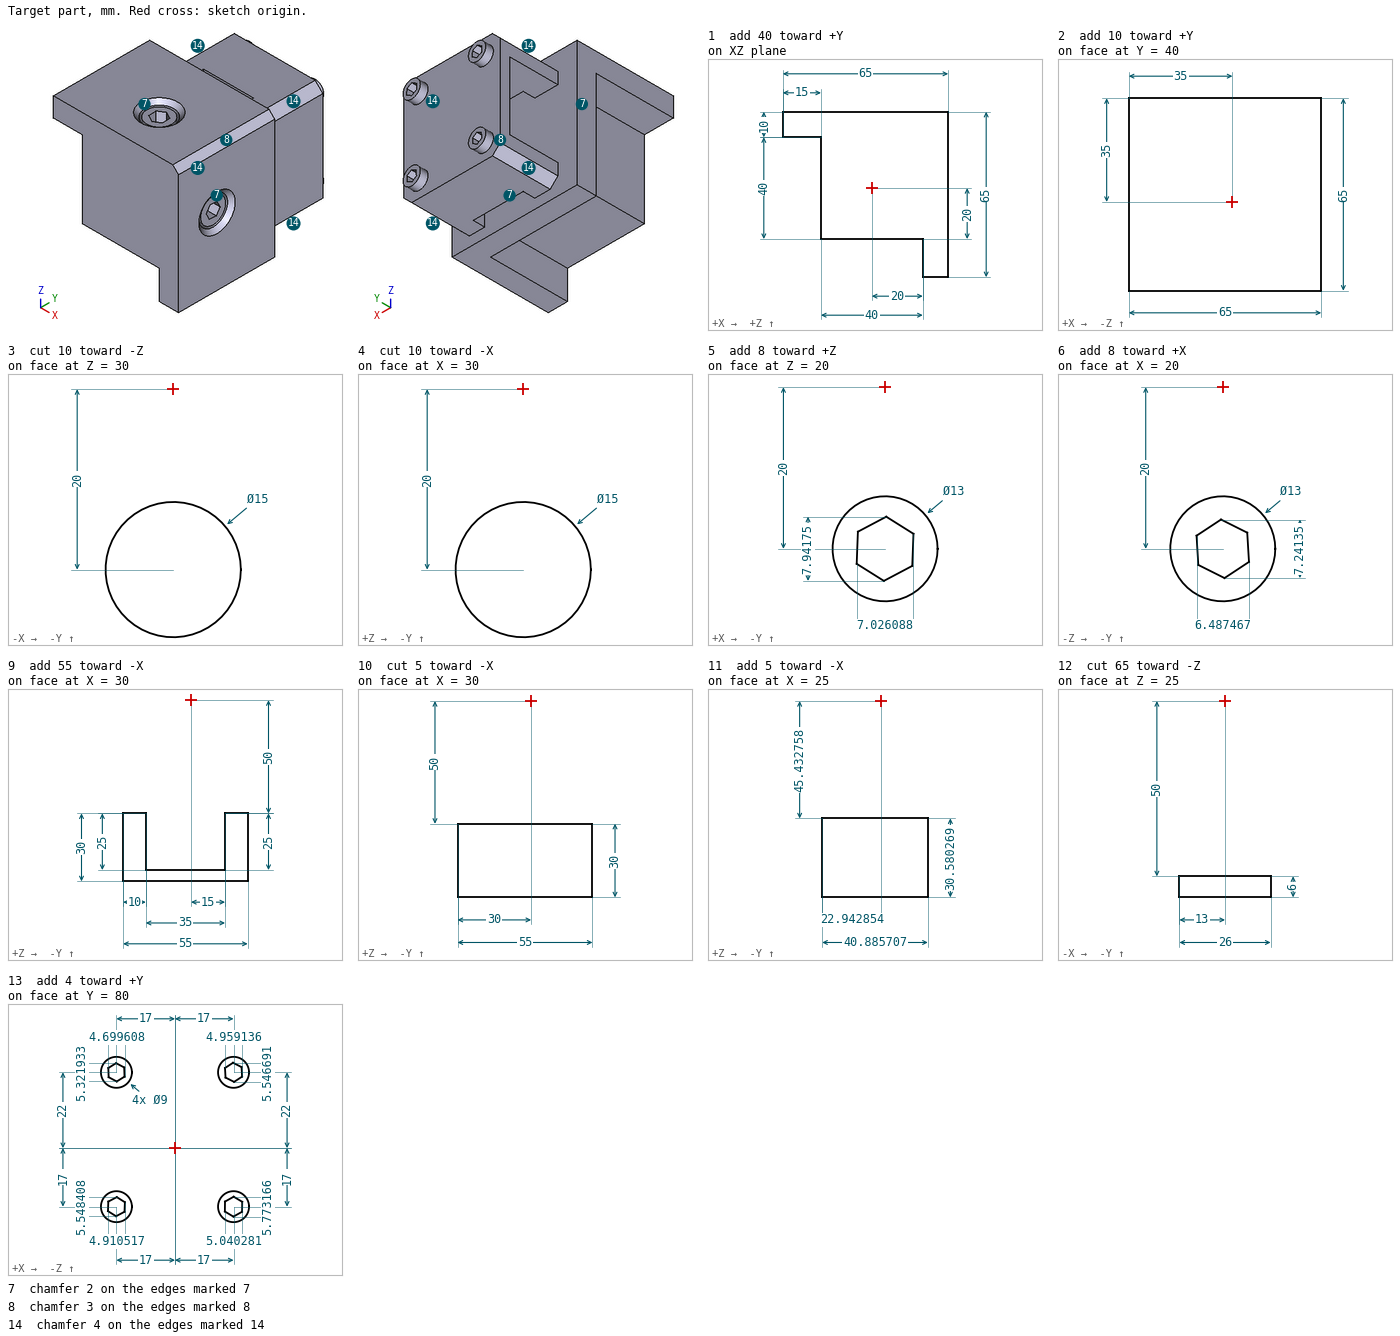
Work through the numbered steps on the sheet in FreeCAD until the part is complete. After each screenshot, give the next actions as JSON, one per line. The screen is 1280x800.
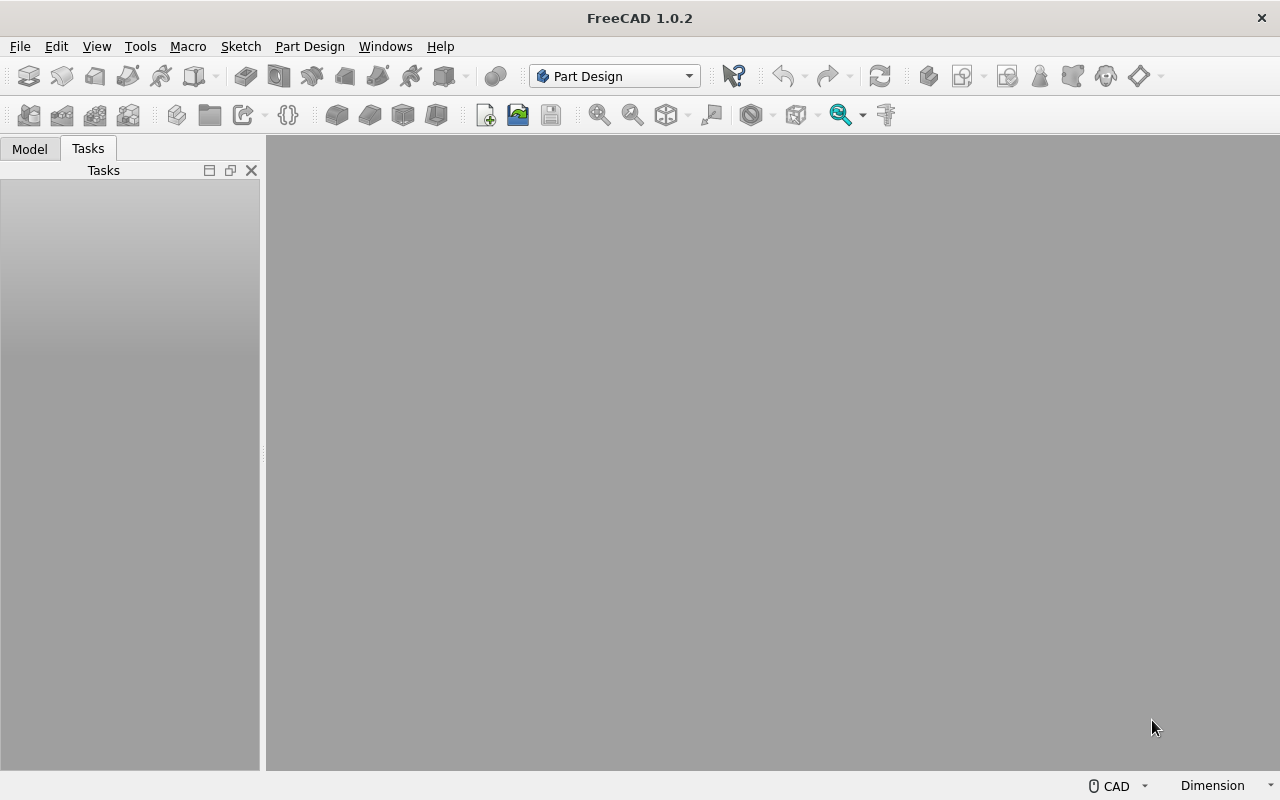
{"action": "left_click", "coordinate": [485, 116]}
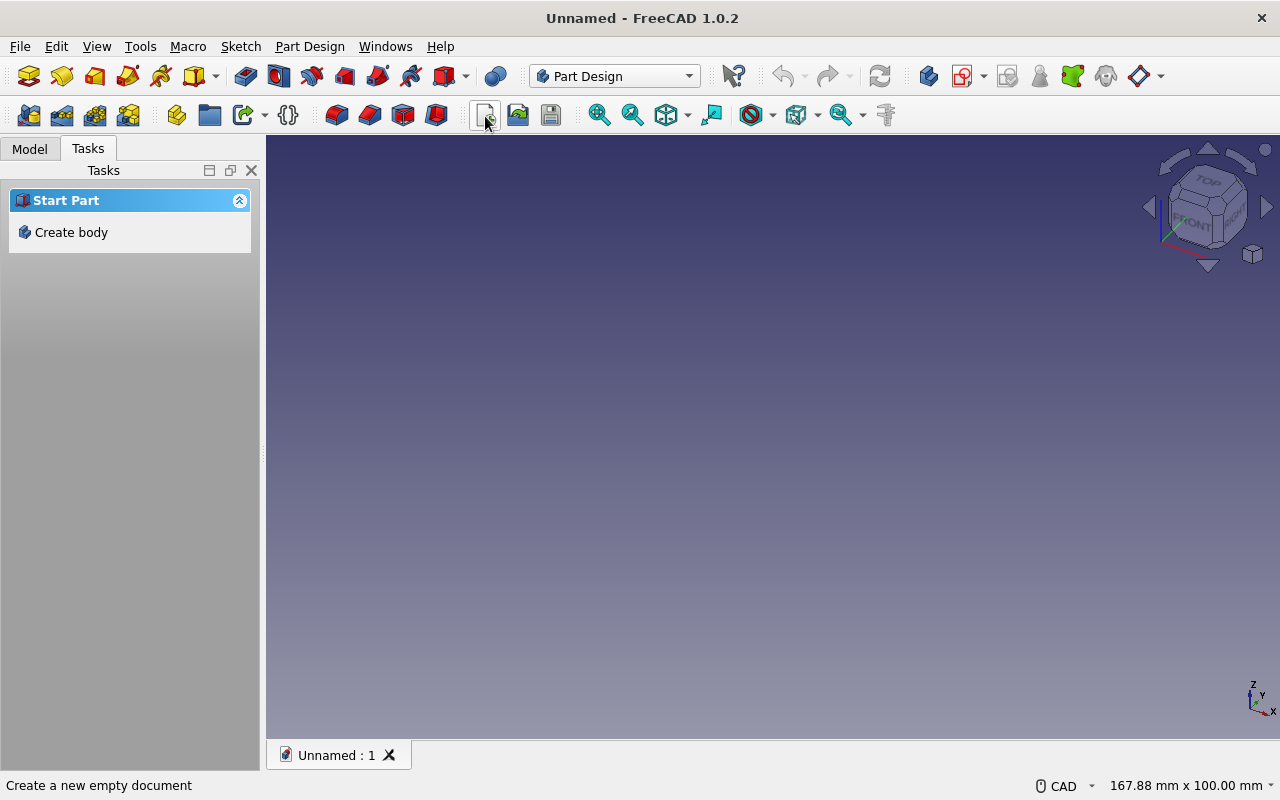
{"action": "left_click", "coordinate": [962, 76]}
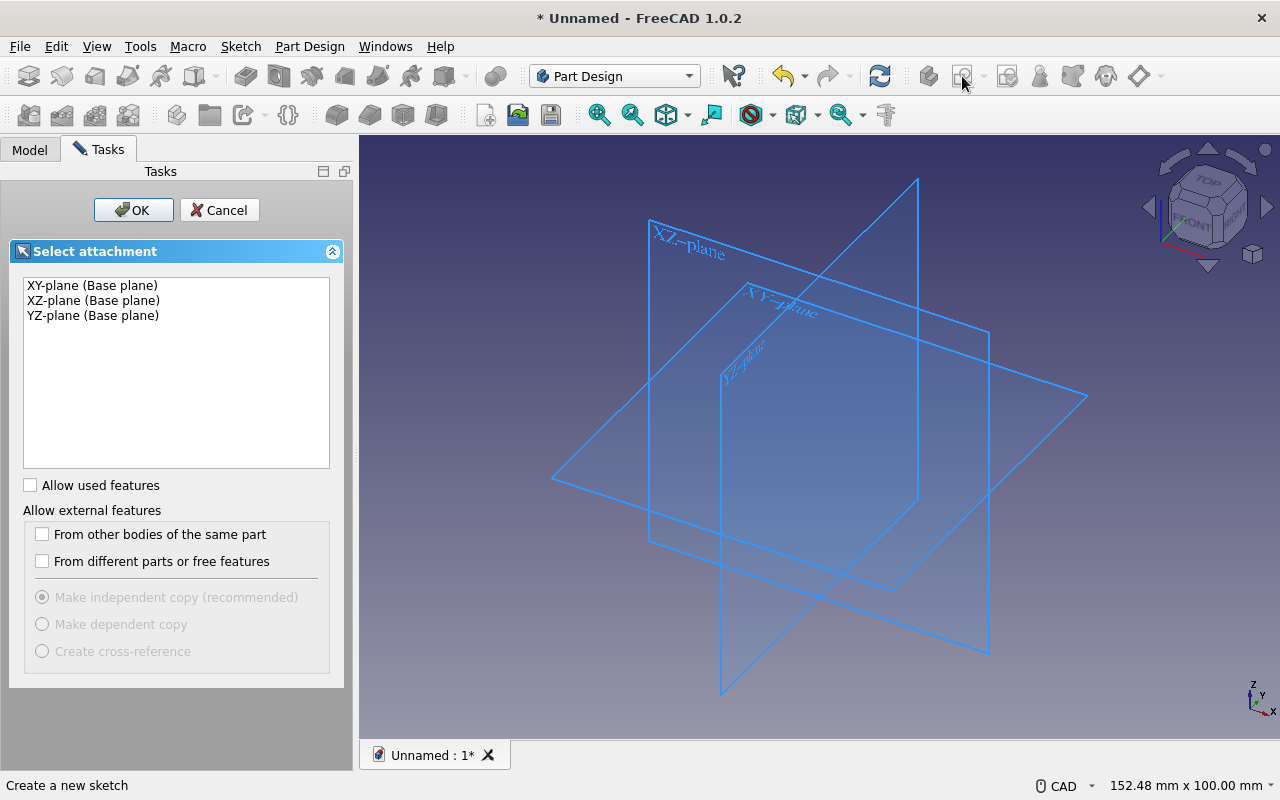
{"action": "left_click", "coordinate": [84, 300]}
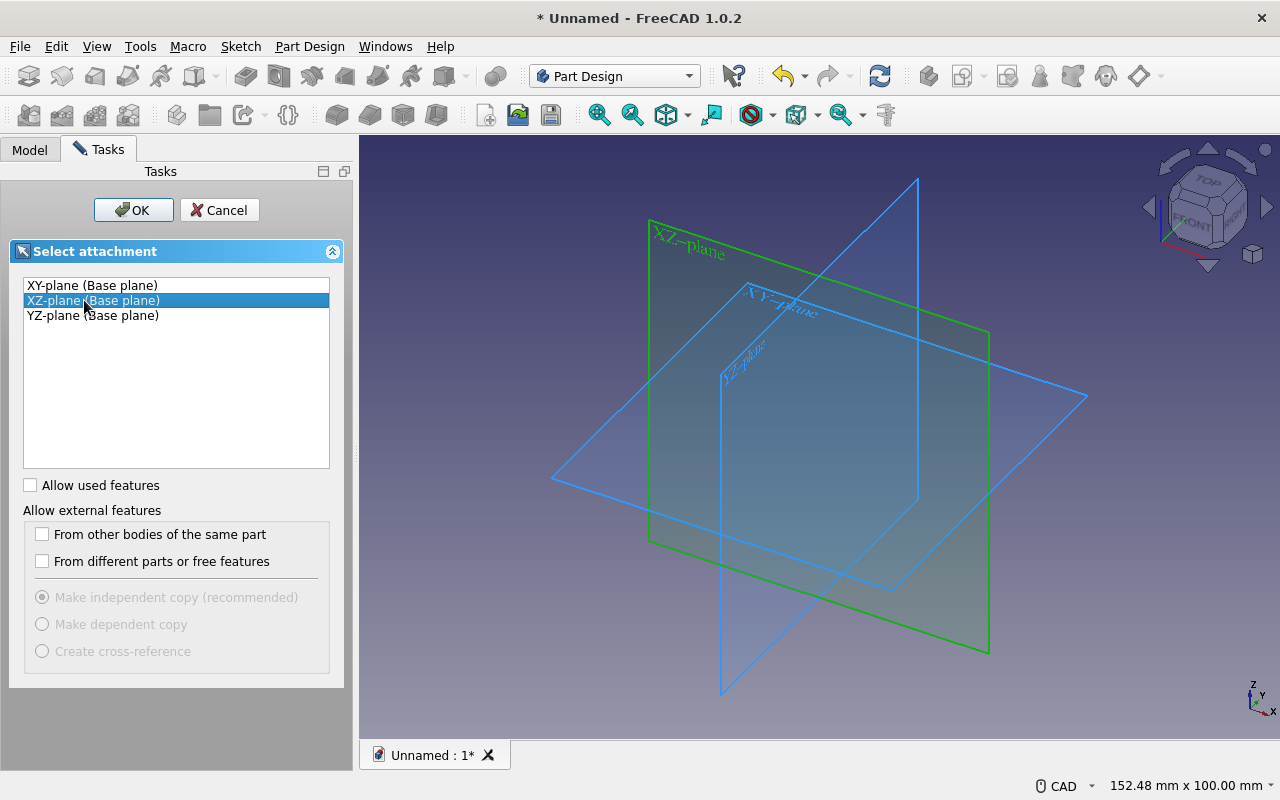
{"action": "left_click", "coordinate": [134, 210]}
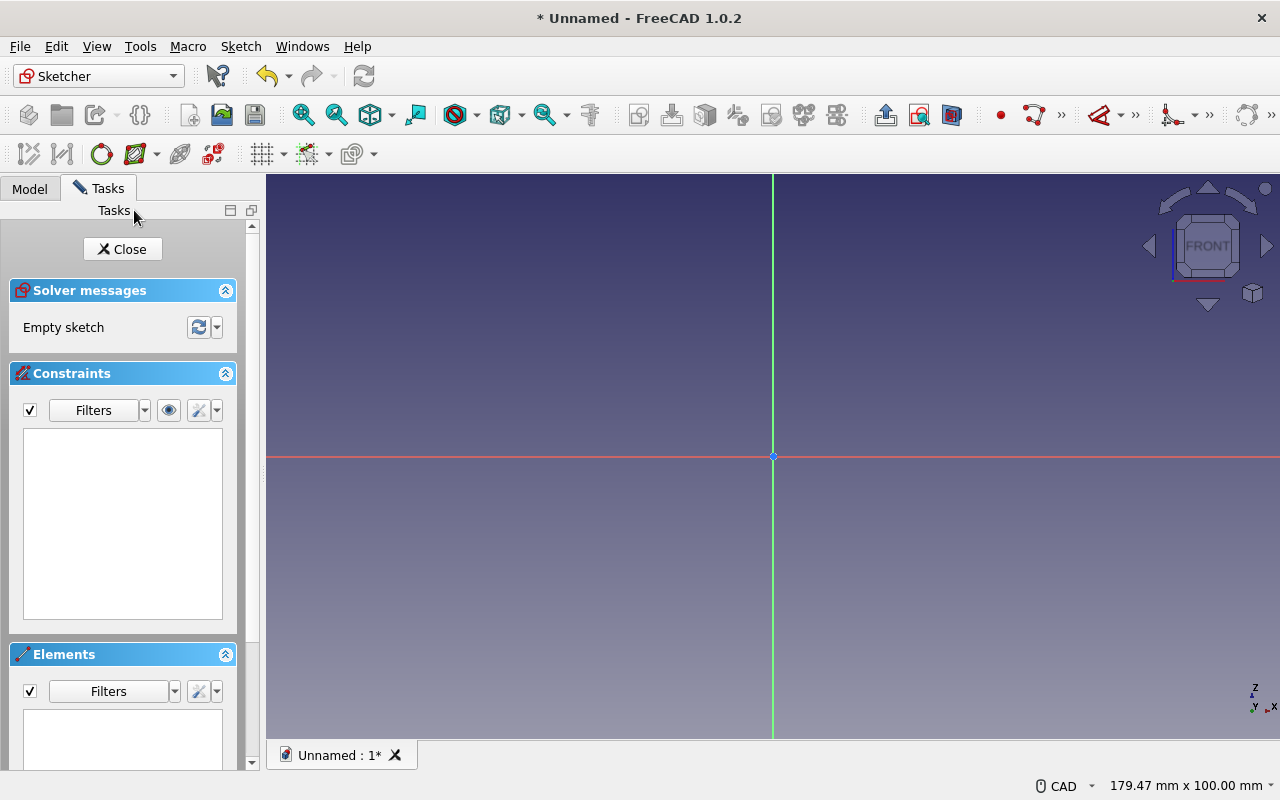
{"action": "left_click", "coordinate": [1034, 116]}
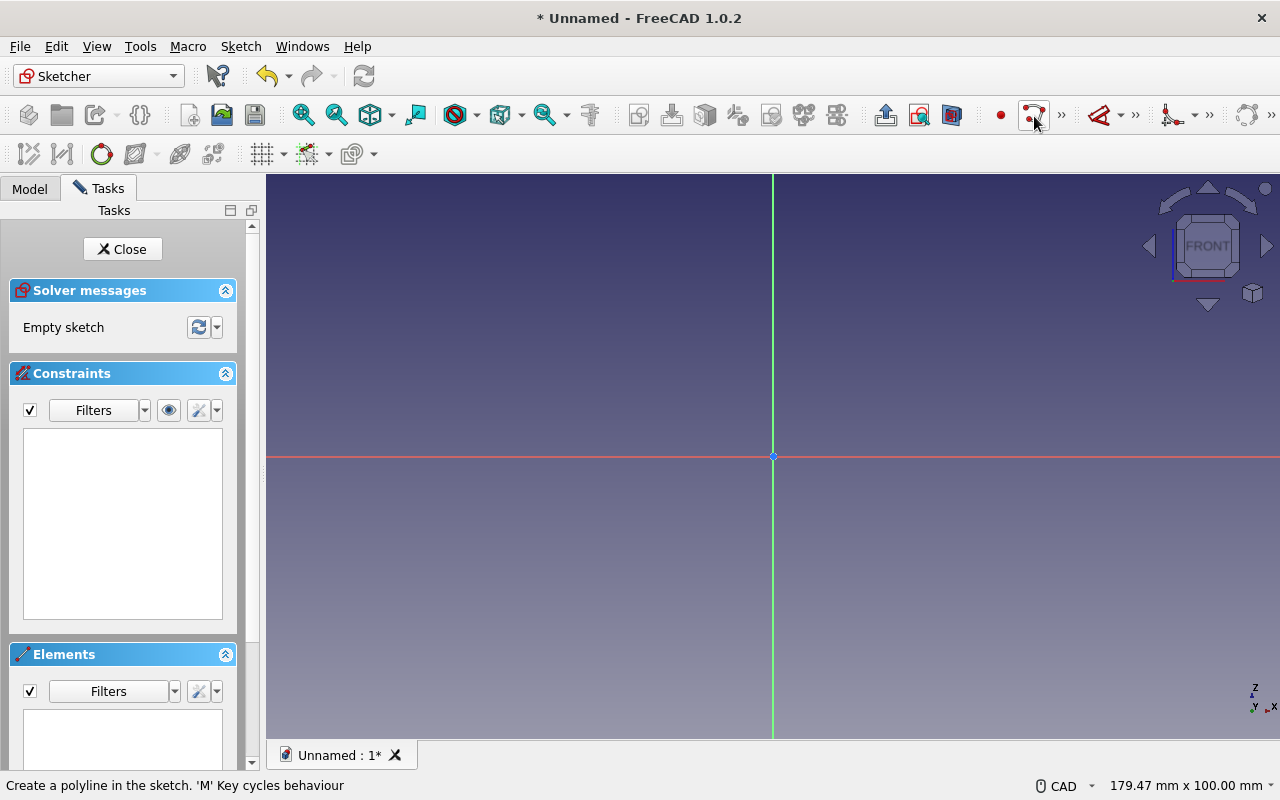
{"action": "left_click", "coordinate": [886, 570]}
{"action": "left_click", "coordinate": [660, 570]}
{"action": "left_click", "coordinate": [660, 344]}
{"action": "left_click", "coordinate": [575, 344]}
{"action": "left_click", "coordinate": [575, 287]}
{"action": "left_click", "coordinate": [942, 287]}
{"action": "left_click", "coordinate": [942, 654]}
{"action": "left_click", "coordinate": [886, 654]}
{"action": "left_click", "coordinate": [886, 571]}
{"action": "key", "text": "Escape"}
{"action": "key", "text": "Escape"}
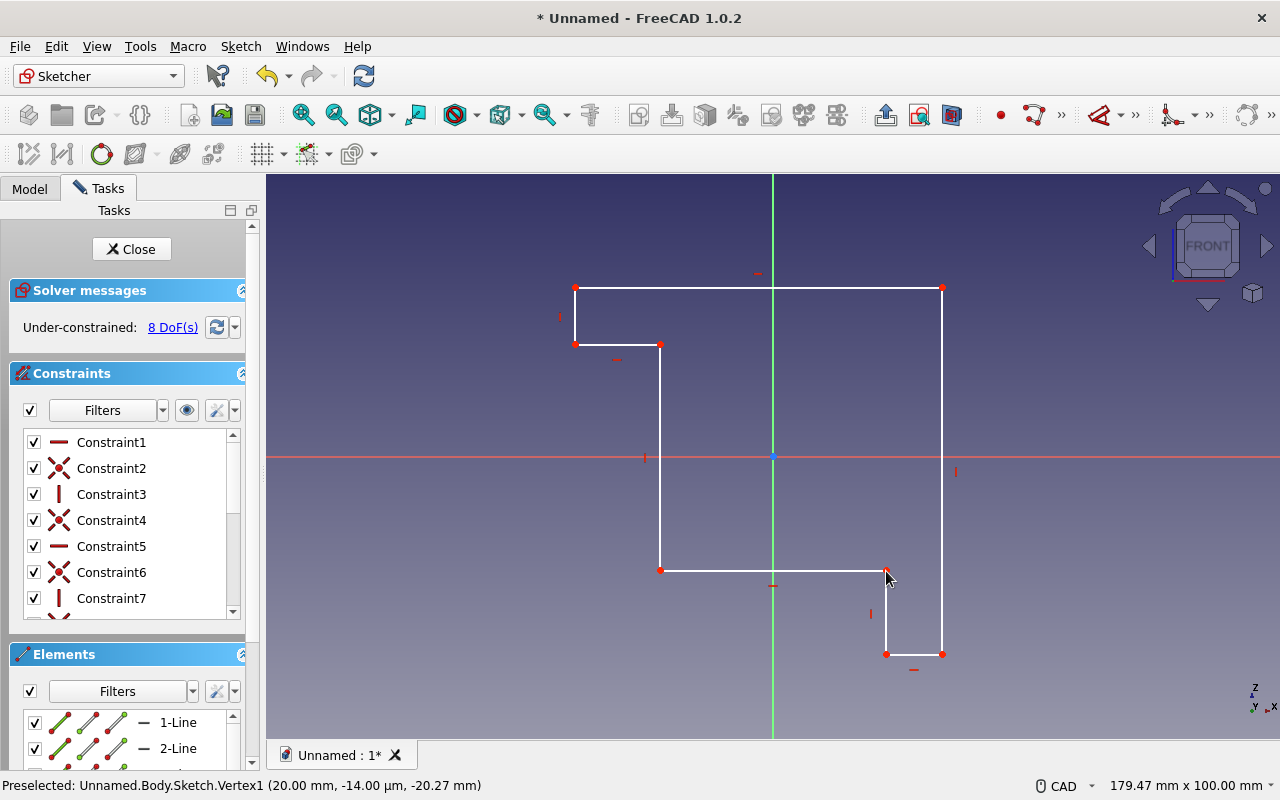
{"action": "left_click", "coordinate": [818, 571]}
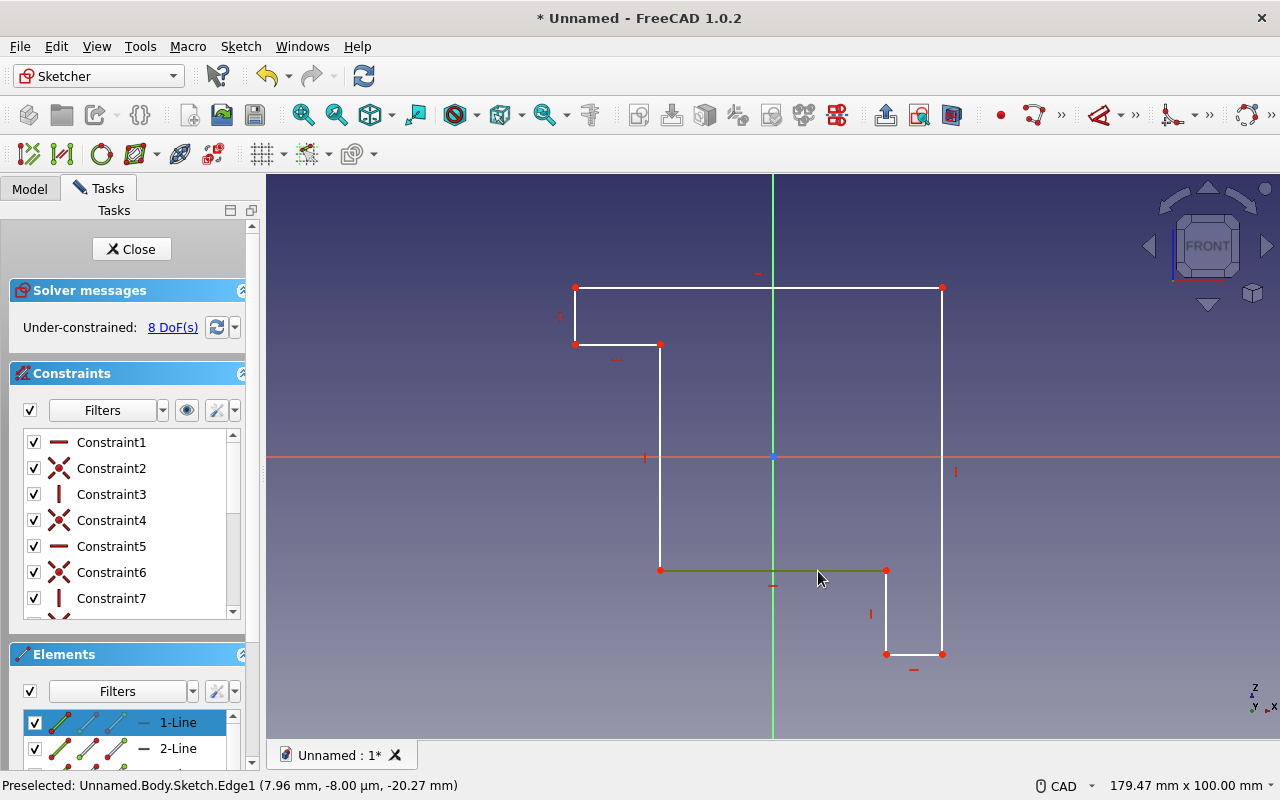
{"action": "key", "text": "l"}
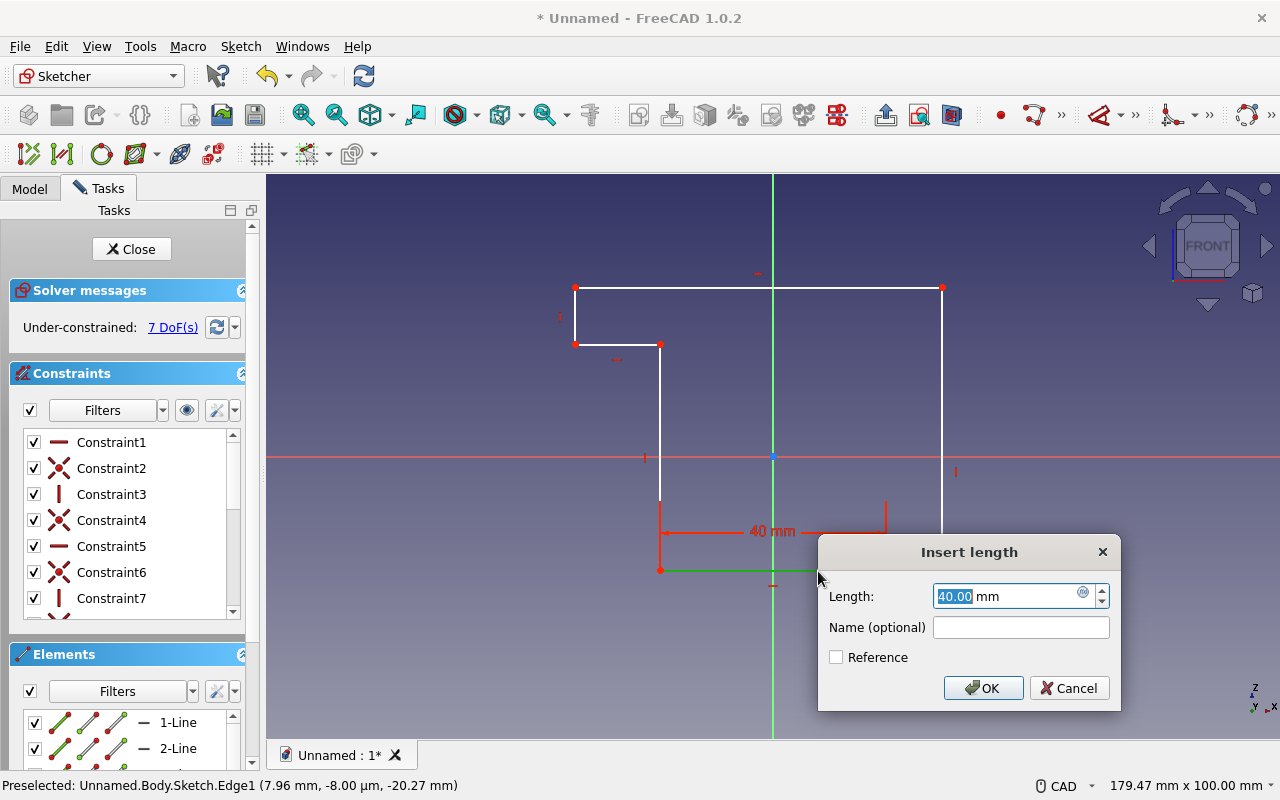
{"action": "type", "text": "40"}
{"action": "key", "text": "Return"}